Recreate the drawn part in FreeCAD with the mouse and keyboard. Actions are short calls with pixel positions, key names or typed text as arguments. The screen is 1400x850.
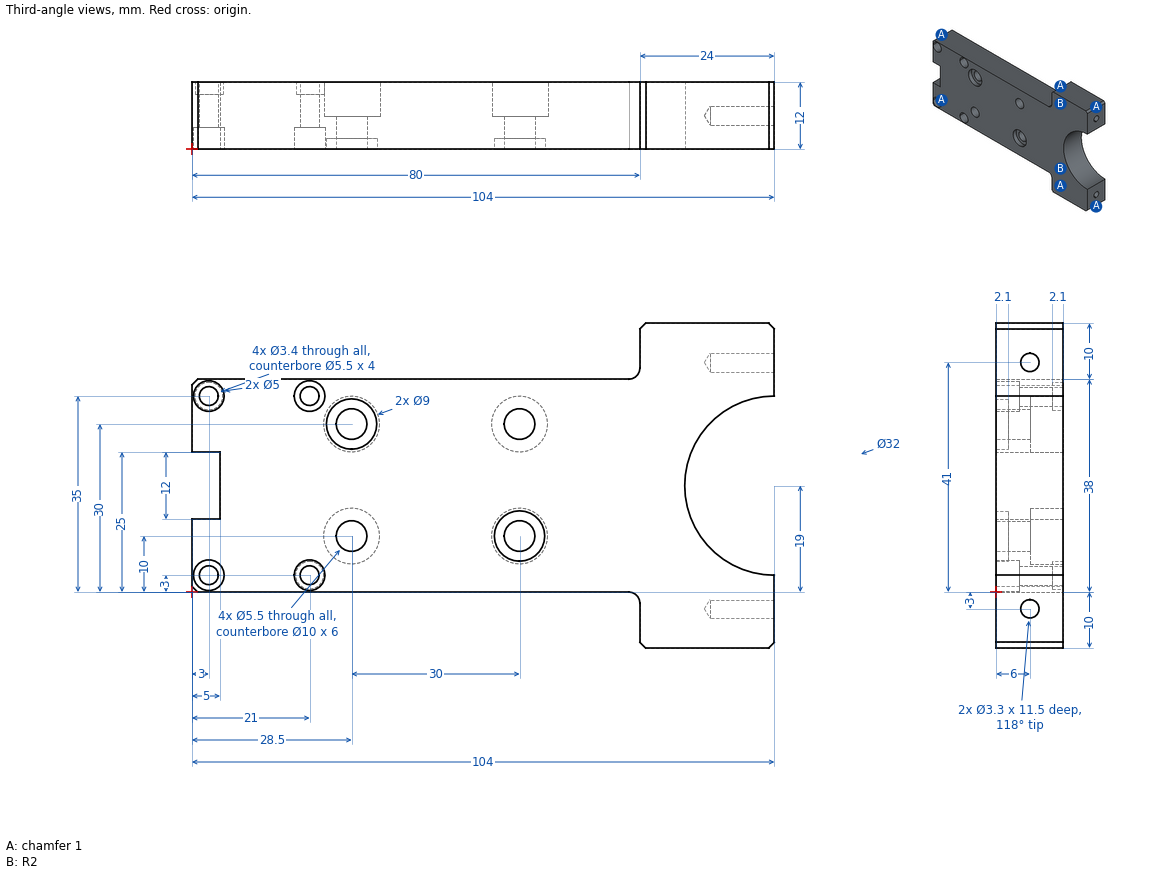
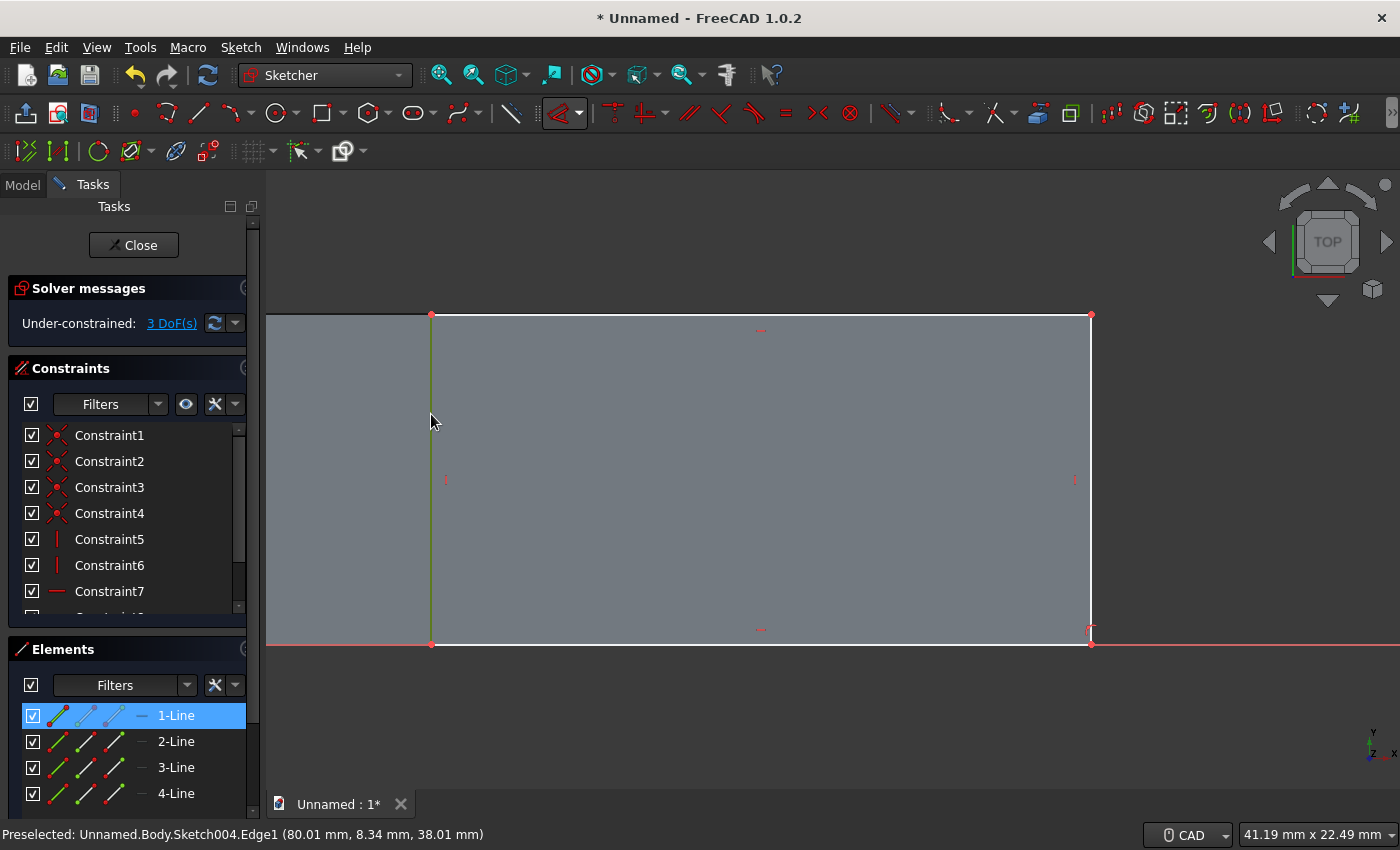
click(582, 114)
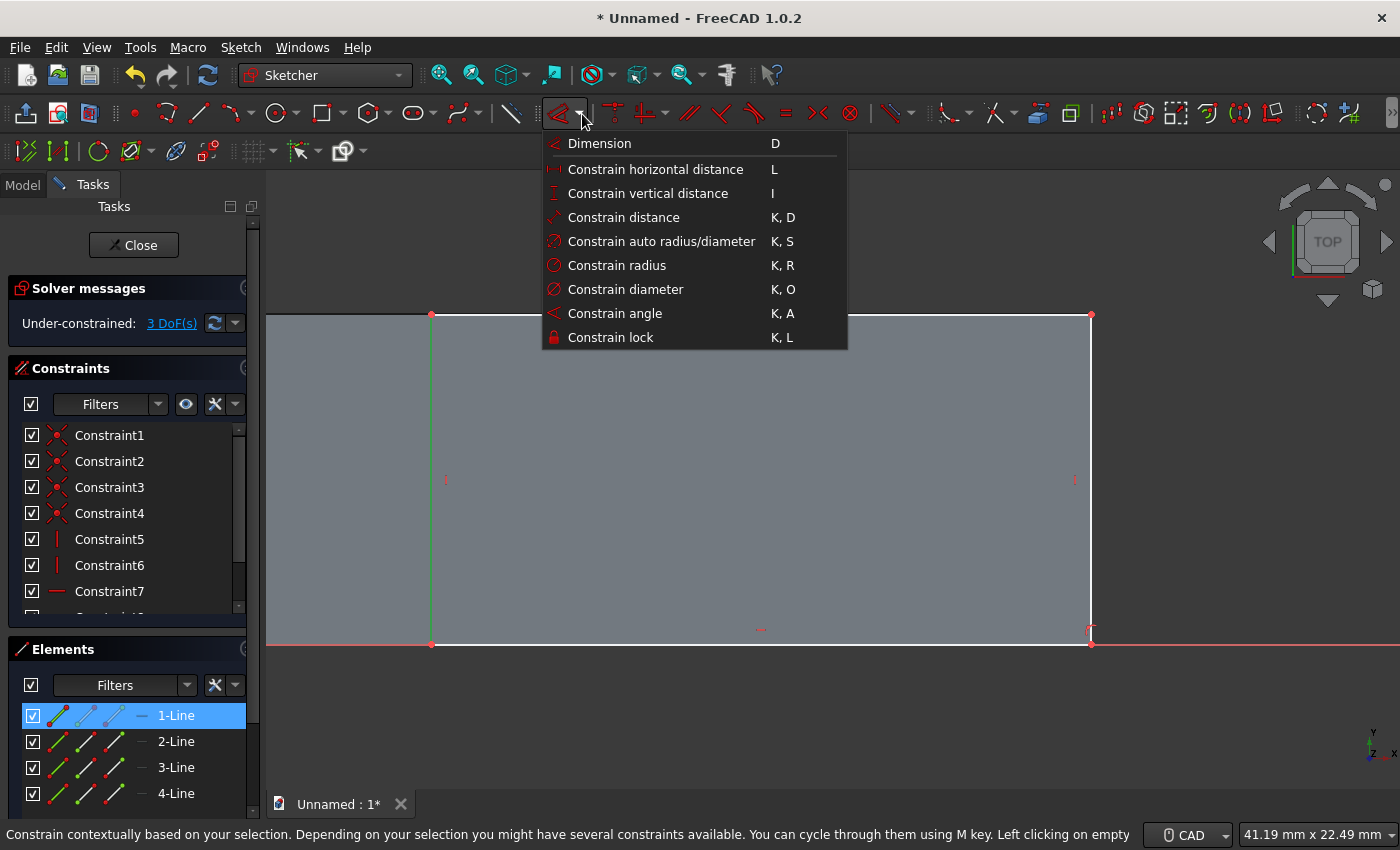
click(695, 193)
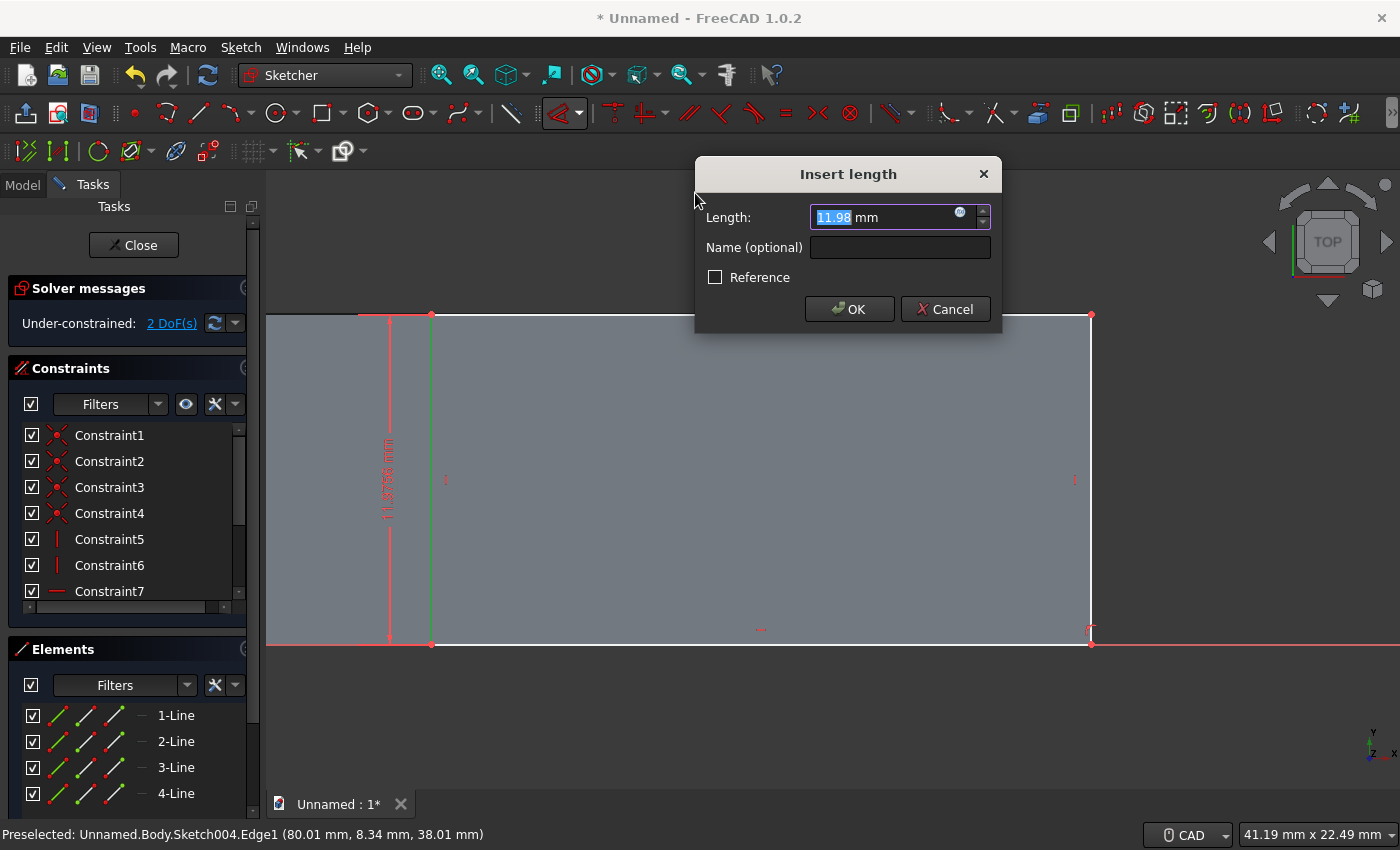
text(12)
key(Return)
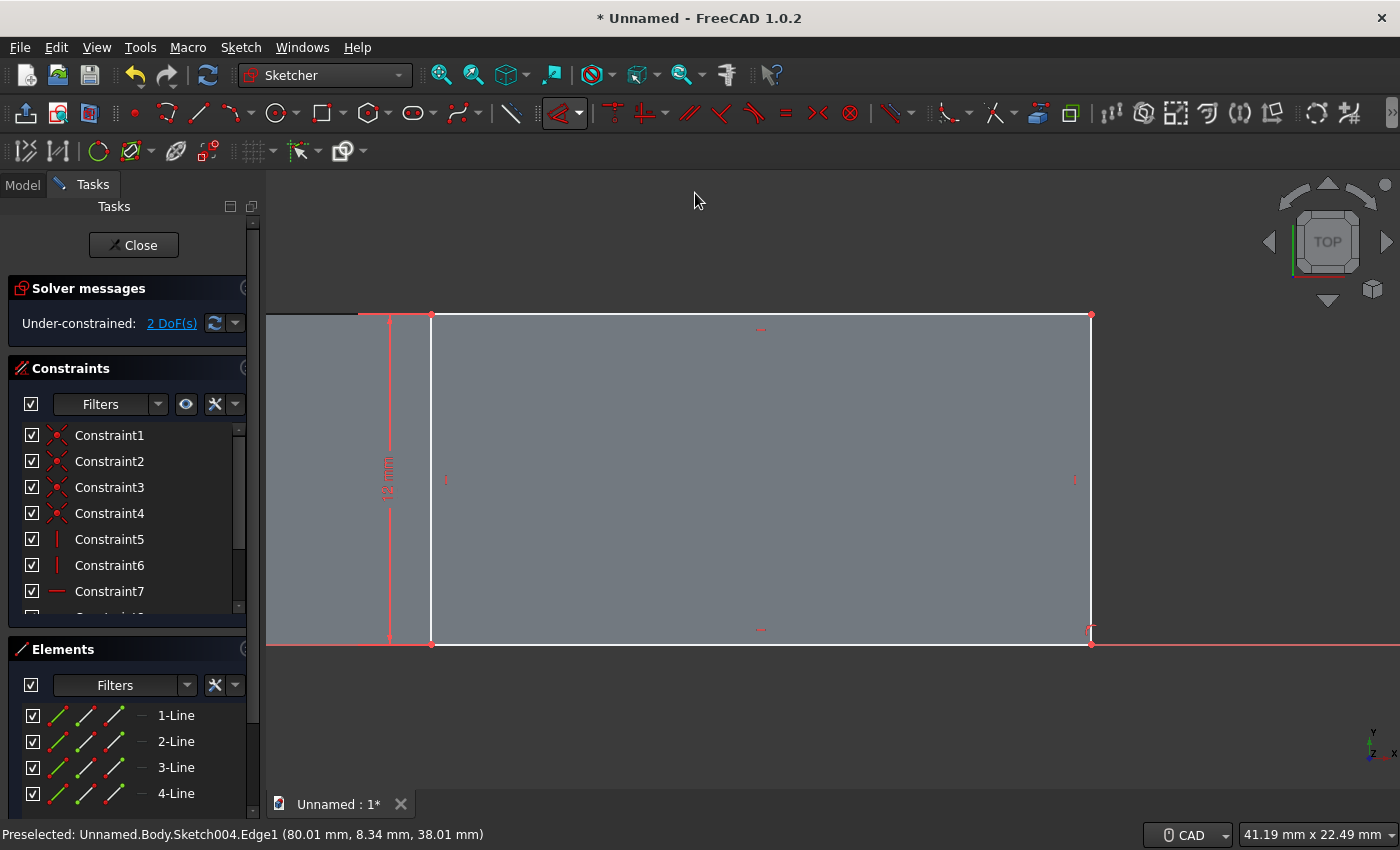
click(629, 645)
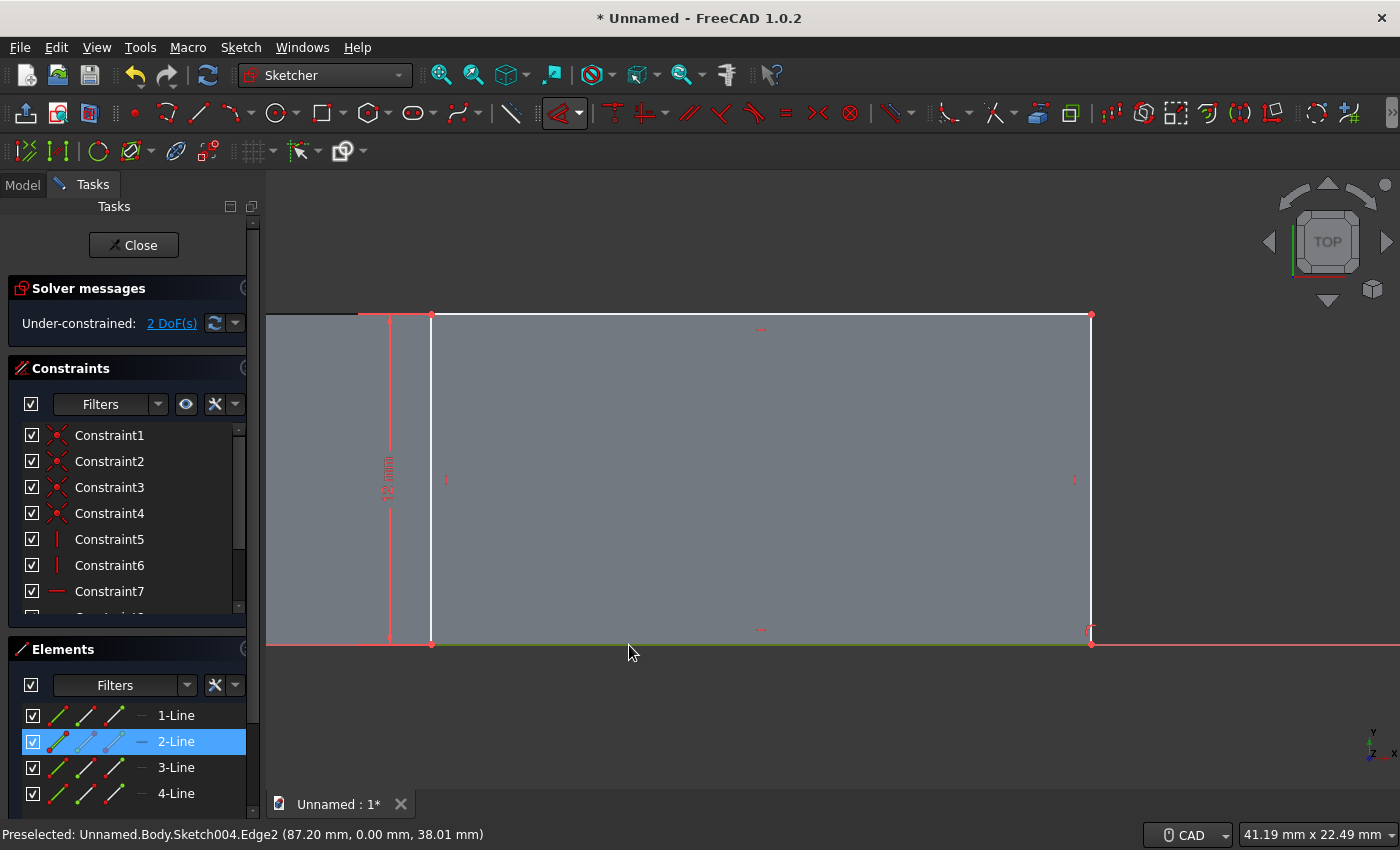
click(582, 114)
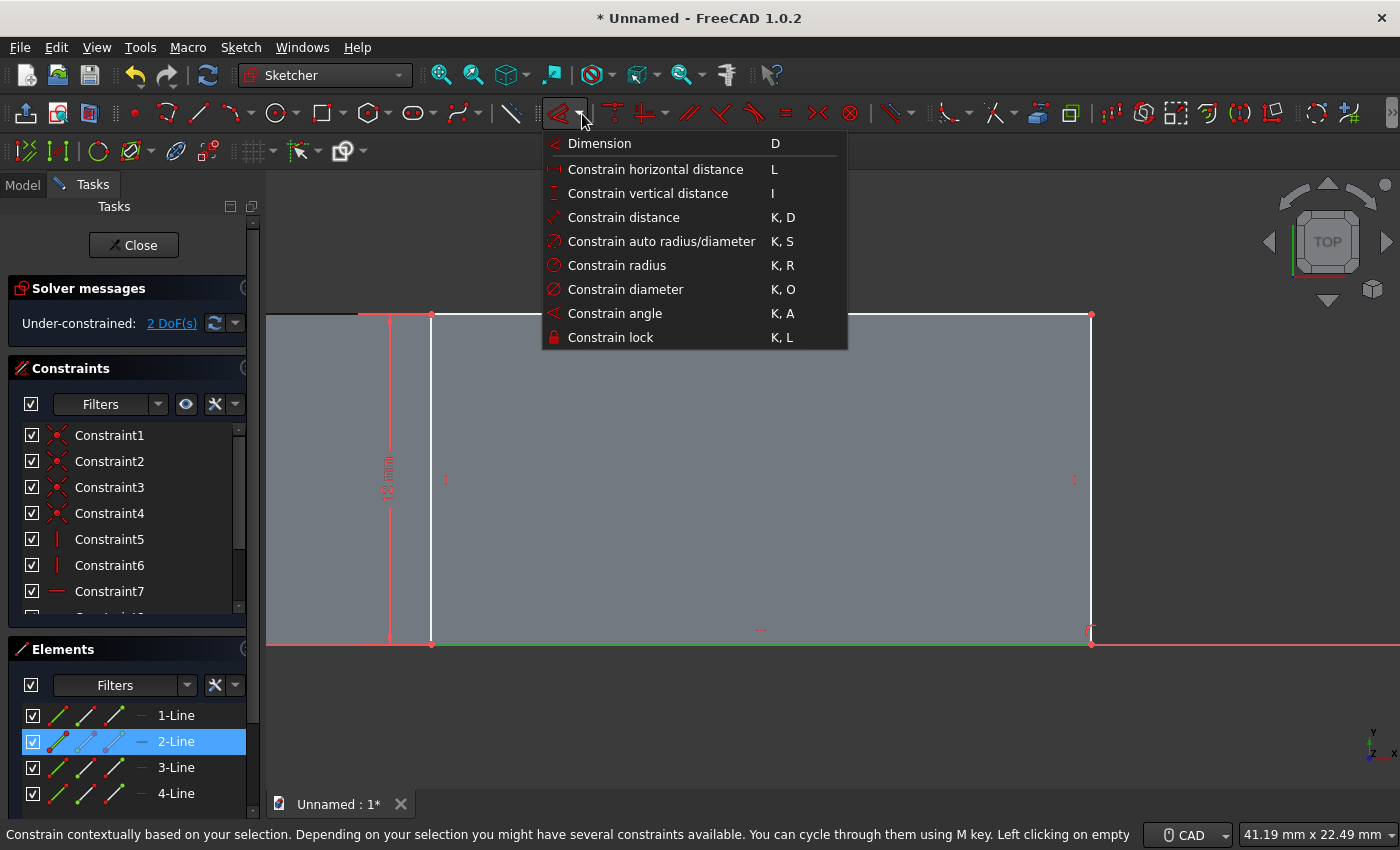
click(695, 169)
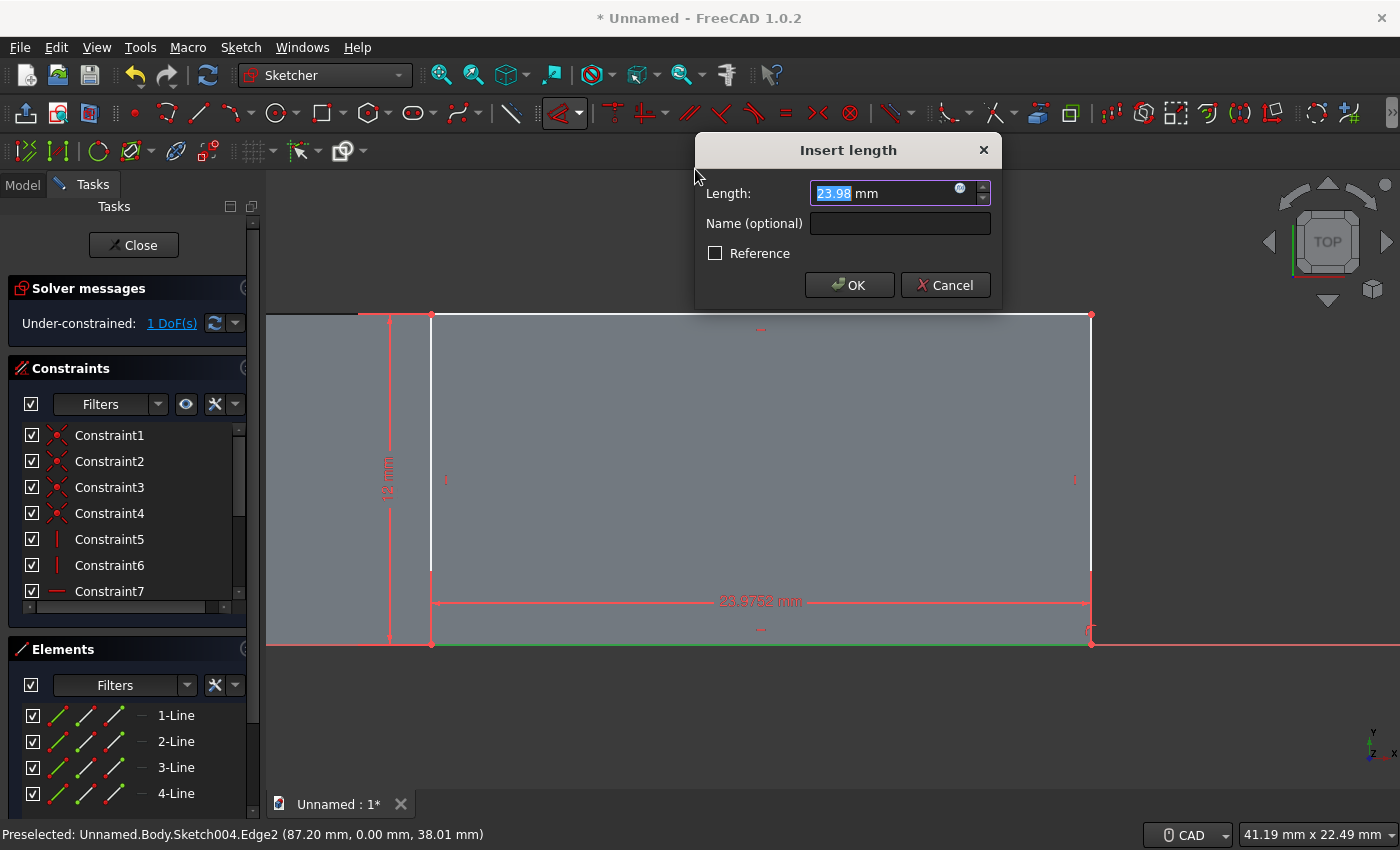
text(24)
key(Return)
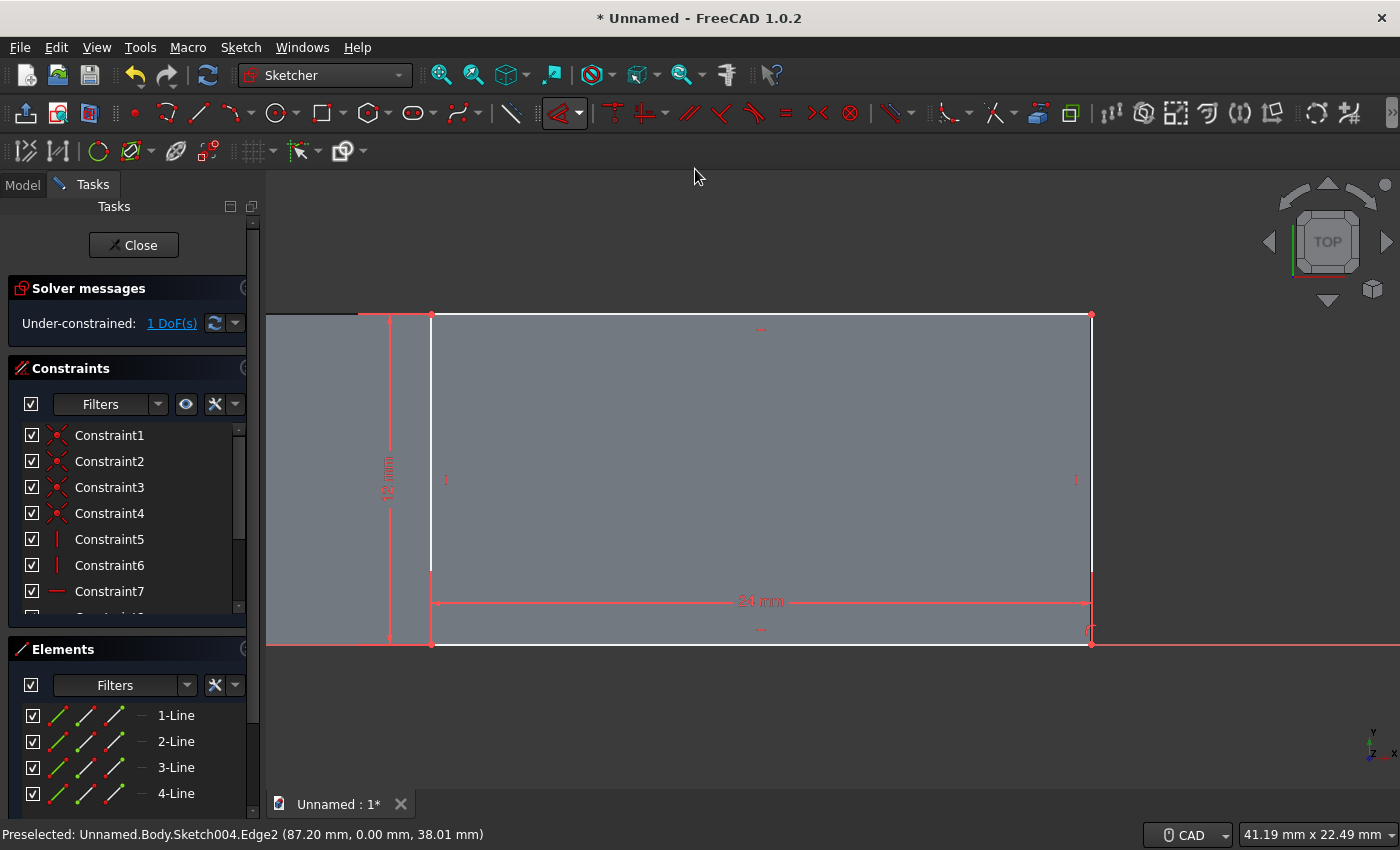
click(431, 314)